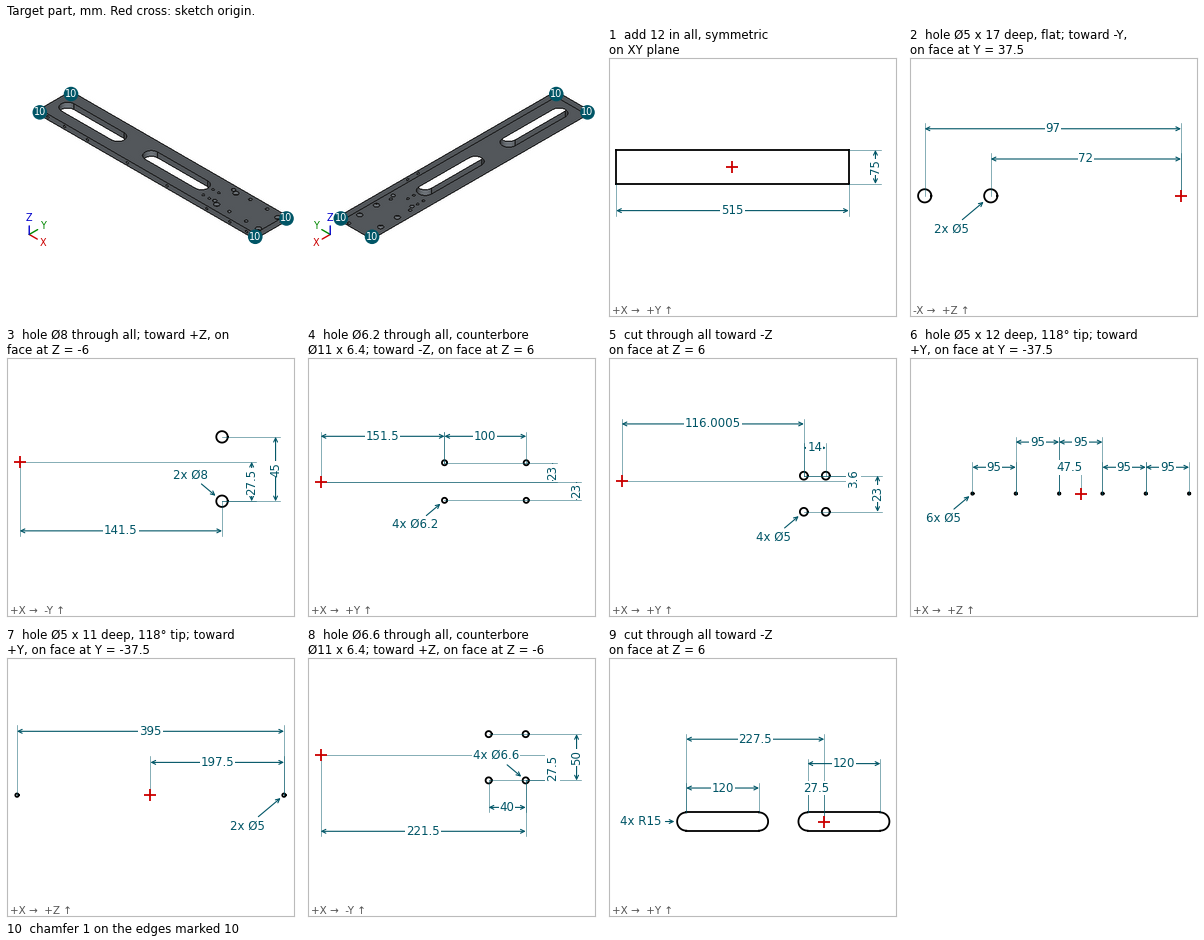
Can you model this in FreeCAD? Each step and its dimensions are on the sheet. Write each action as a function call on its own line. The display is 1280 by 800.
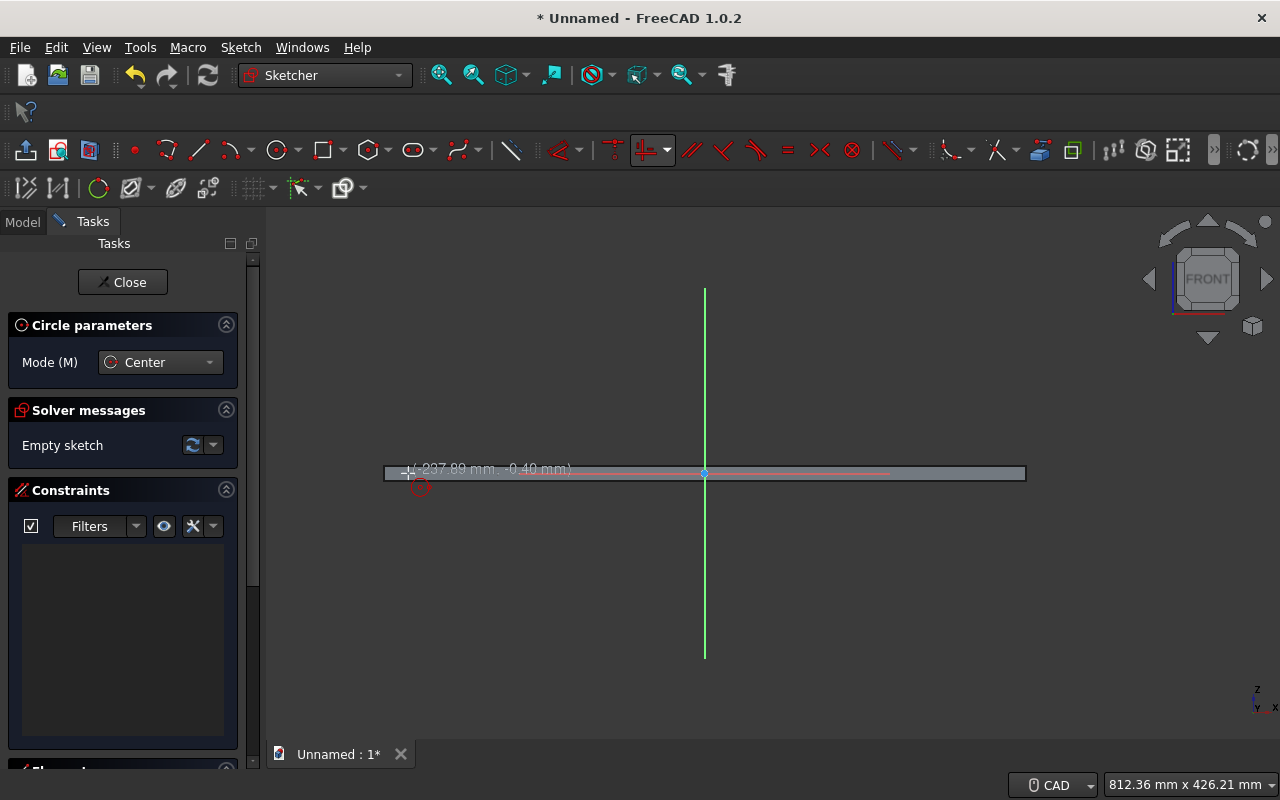
click(408, 473)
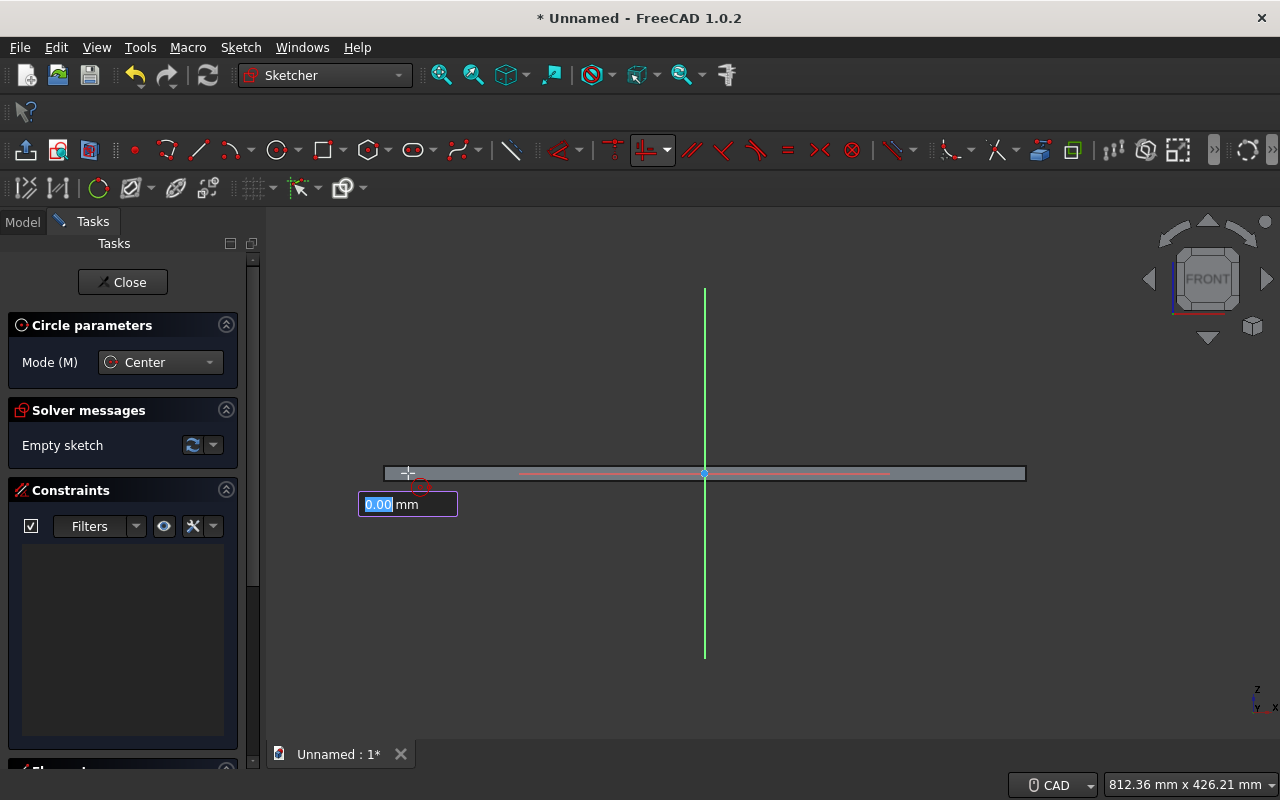
scroll(407, 476, up, 9)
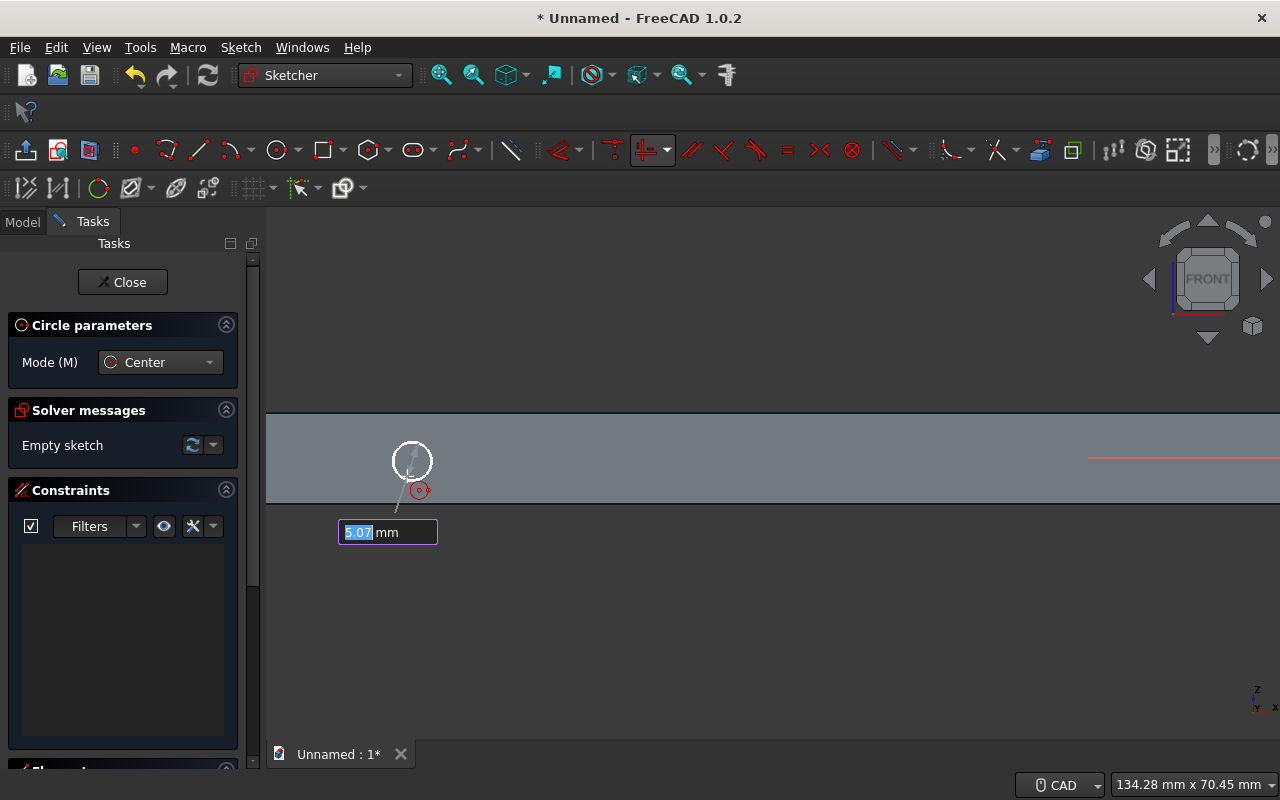
click(409, 476)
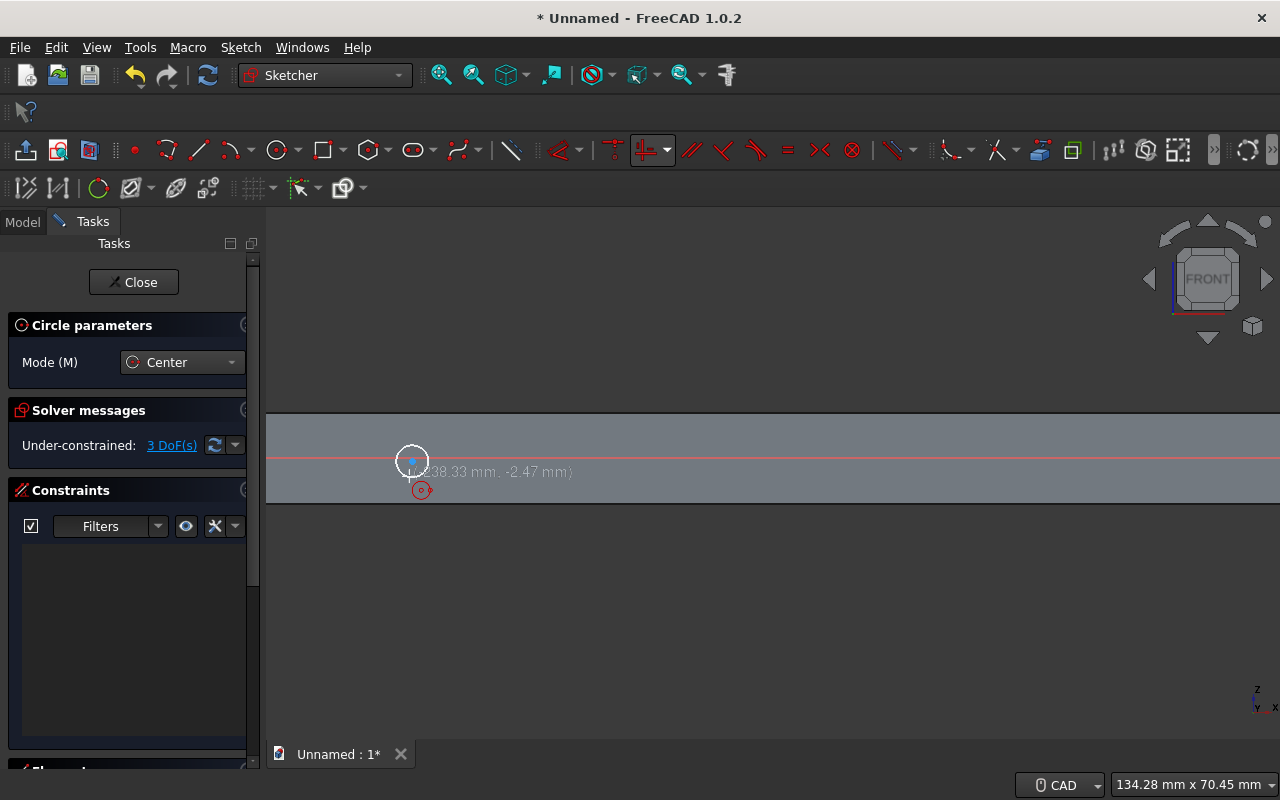
scroll(407, 476, down, 9)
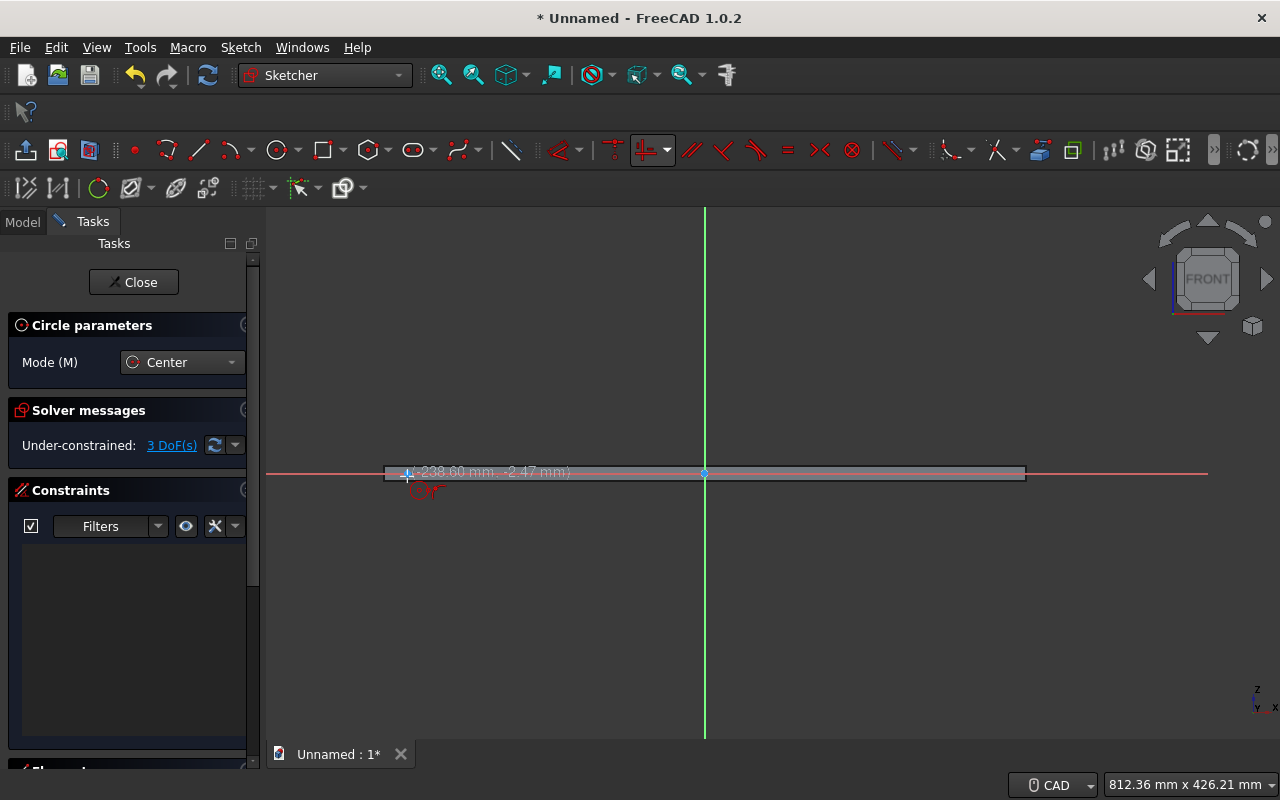
scroll(527, 473, up, 10)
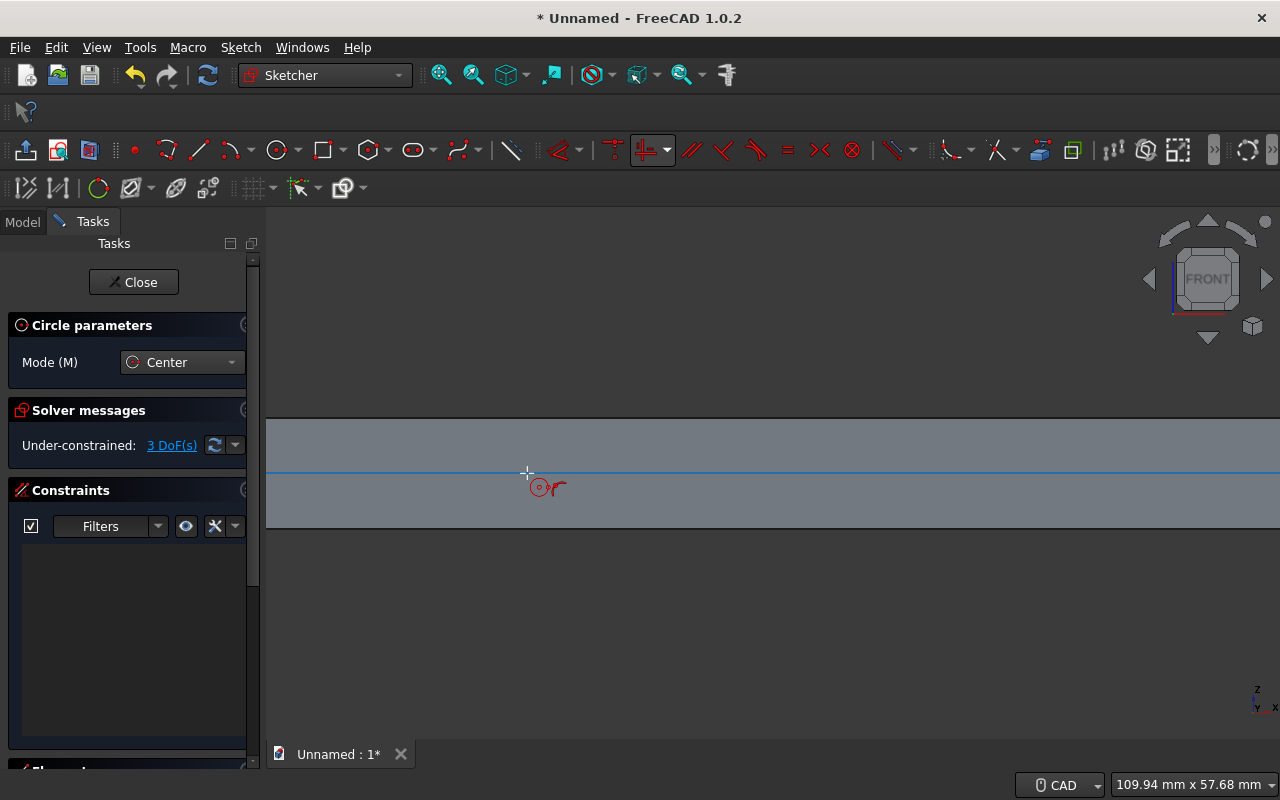
scroll(527, 473, down, 10)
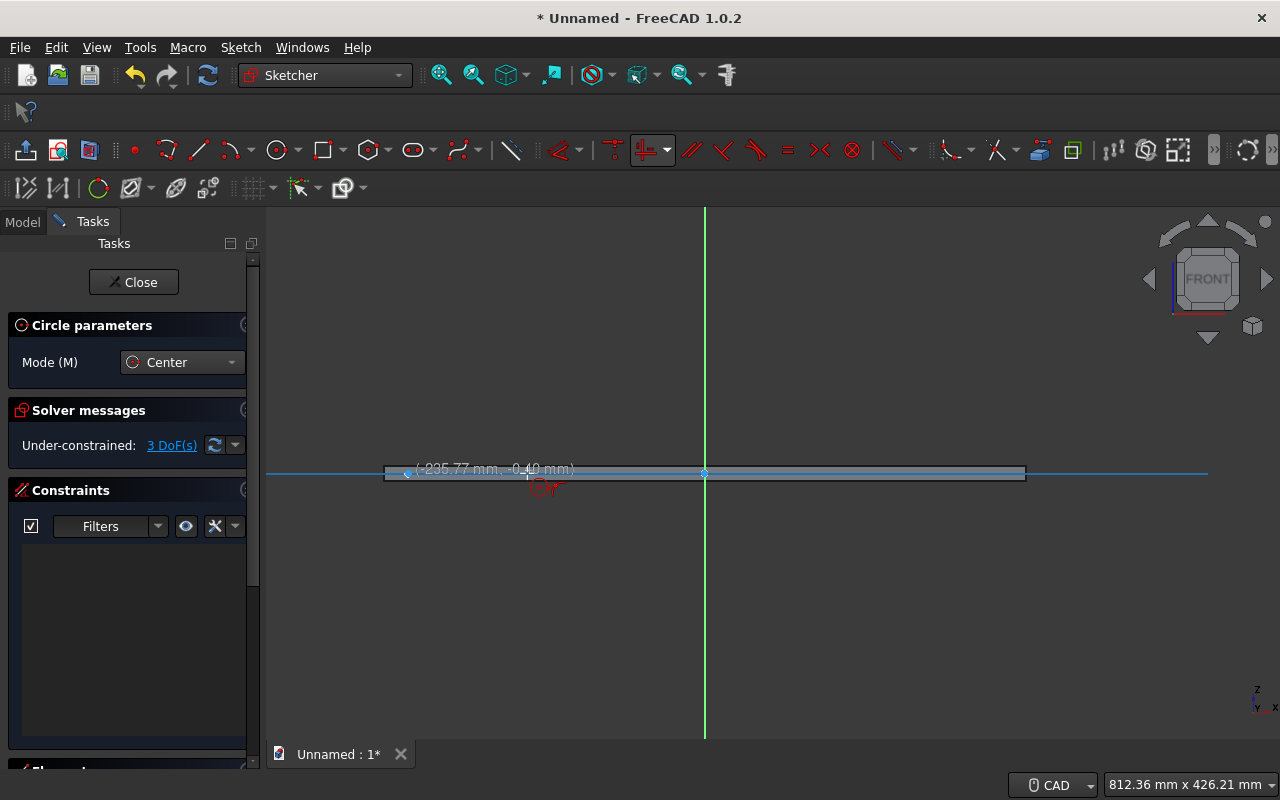
click(527, 473)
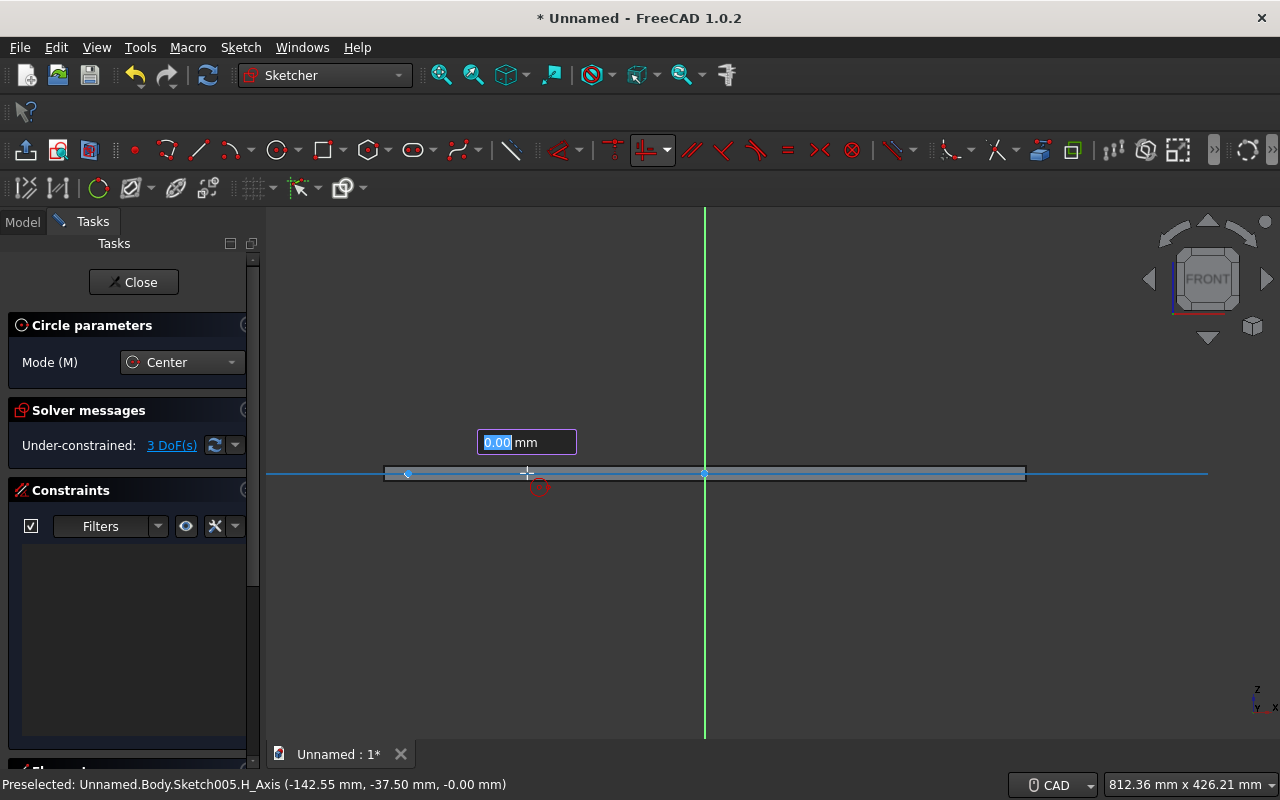
scroll(526, 476, up, 9)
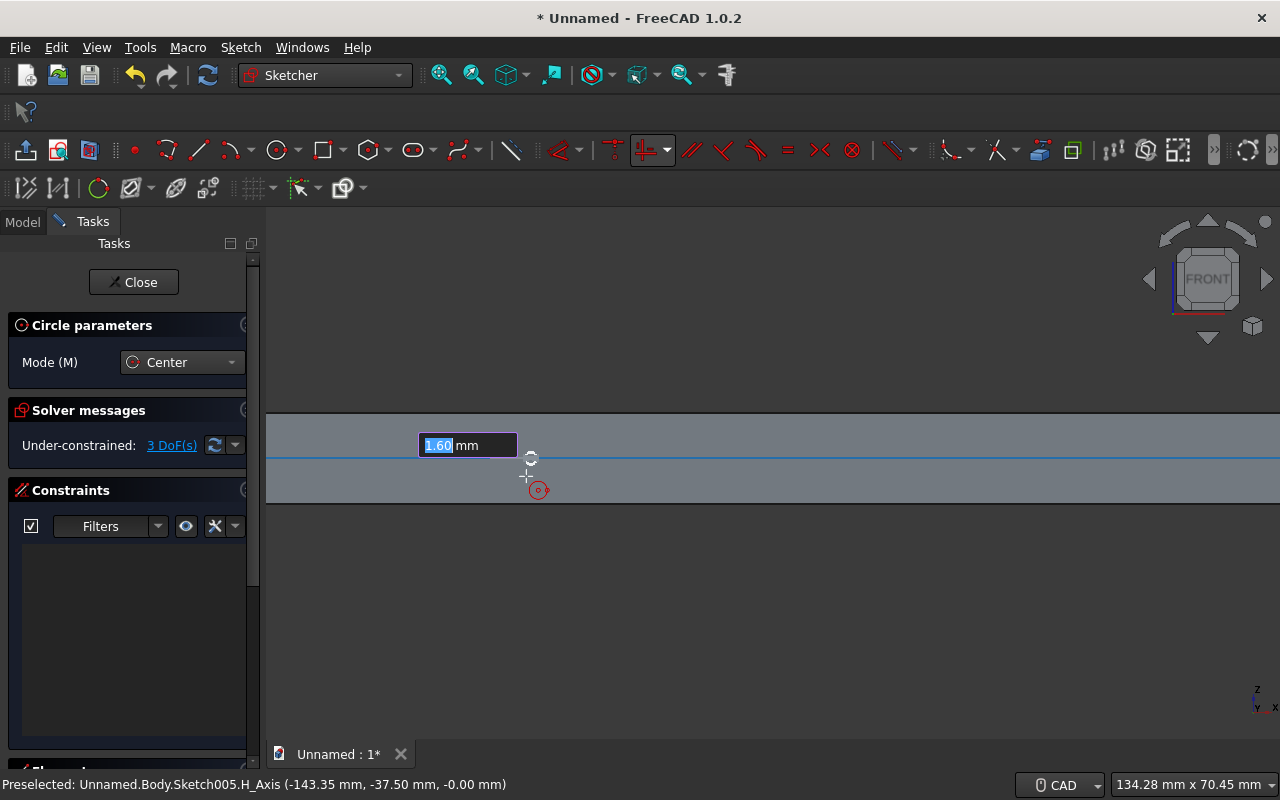
click(525, 476)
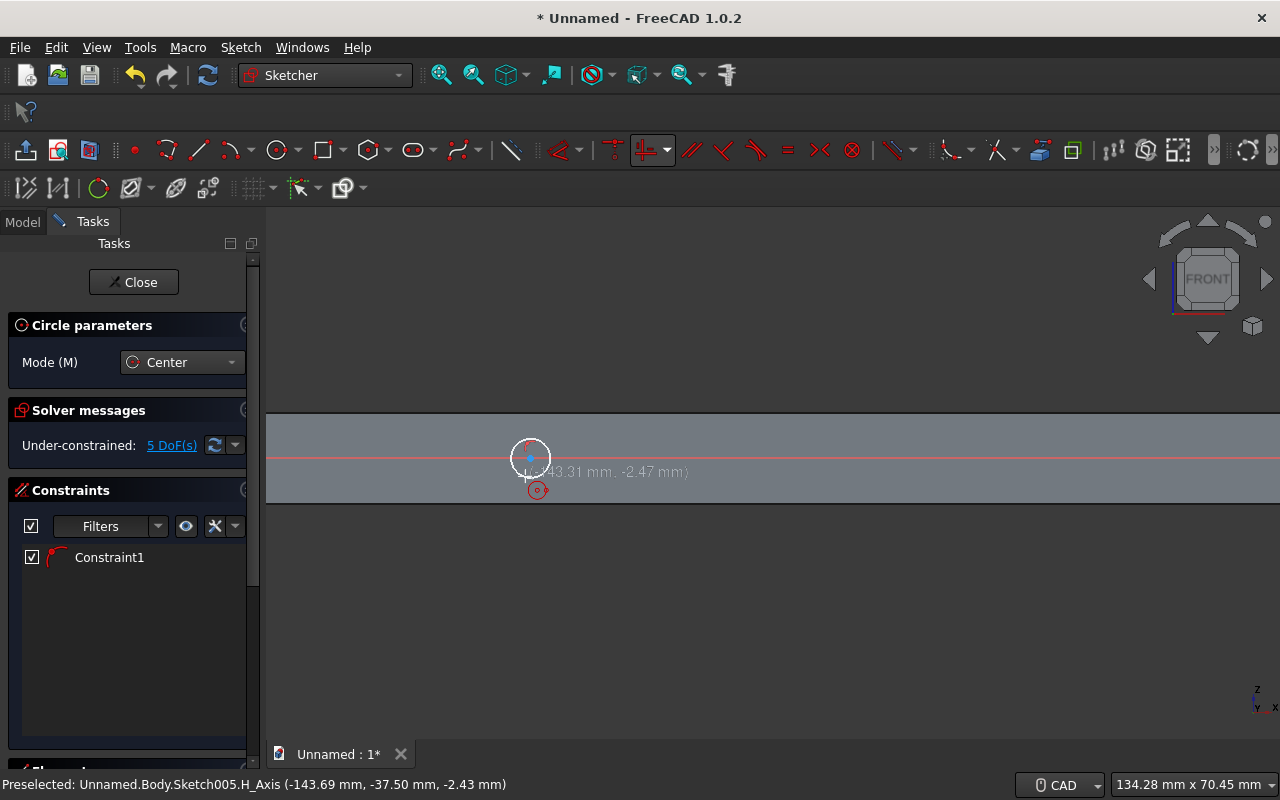
scroll(526, 476, down, 9)